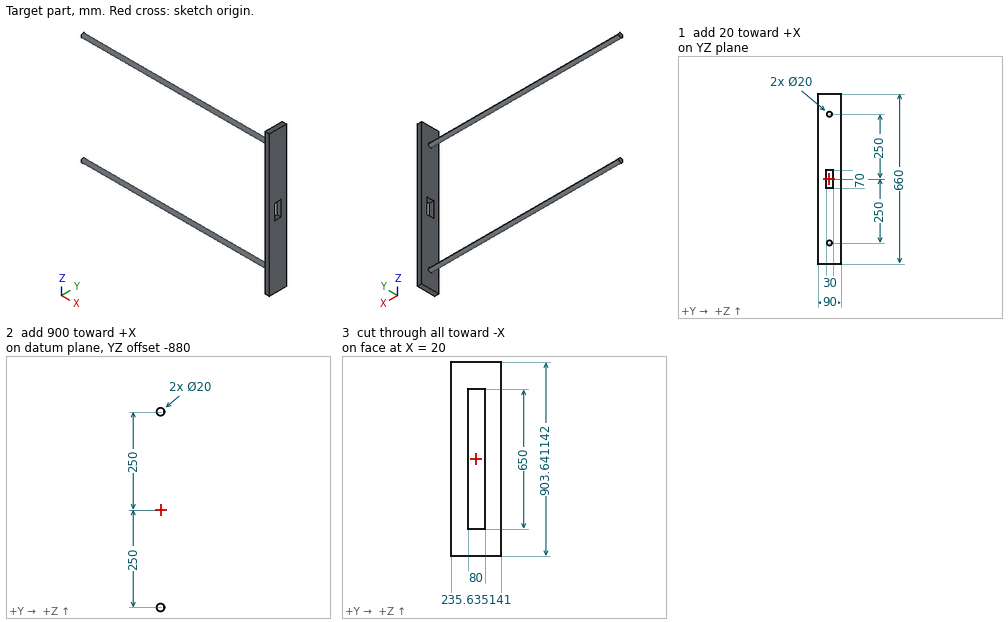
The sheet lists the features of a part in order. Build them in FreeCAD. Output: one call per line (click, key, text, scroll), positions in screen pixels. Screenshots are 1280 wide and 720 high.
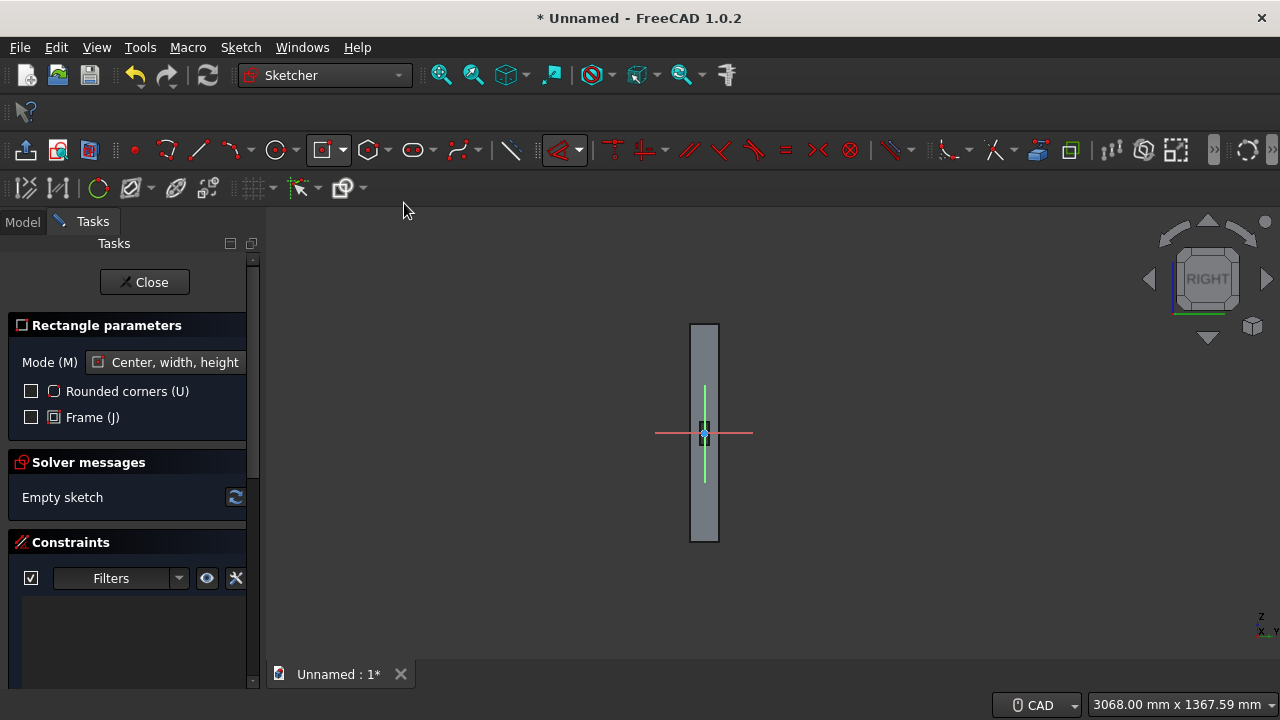
click(705, 433)
click(743, 284)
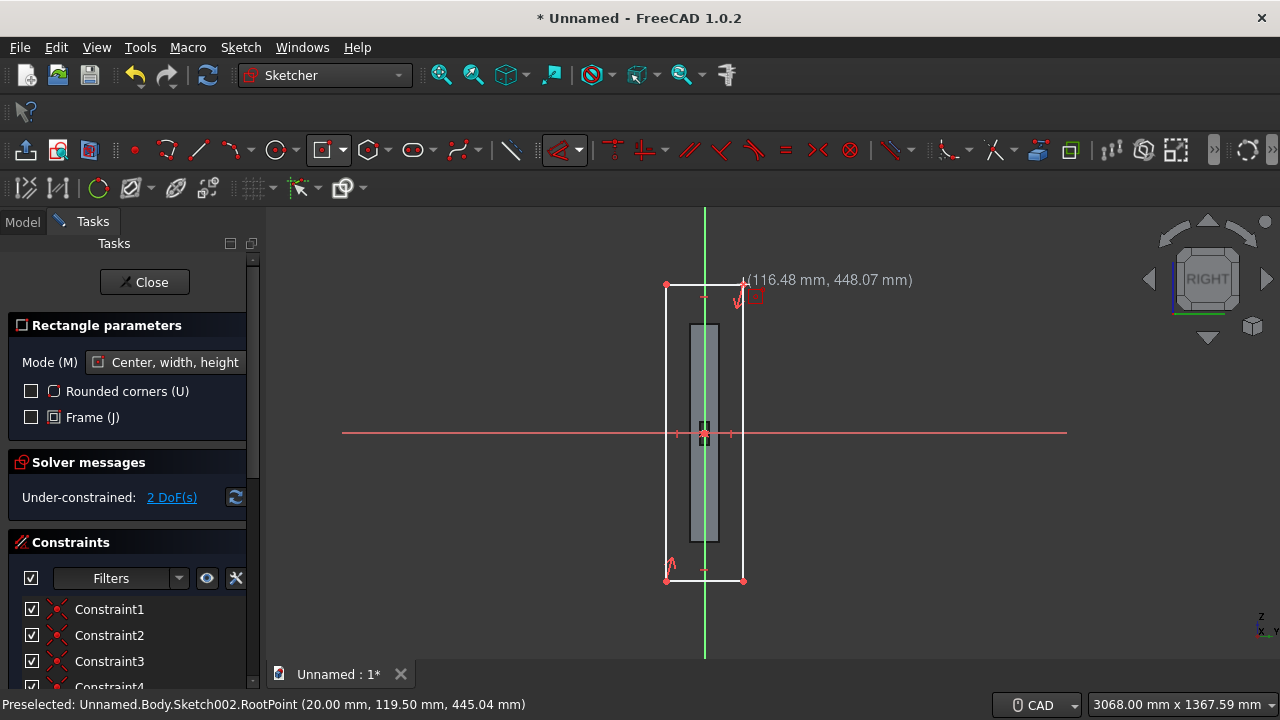
click(705, 433)
click(718, 326)
key(Escape)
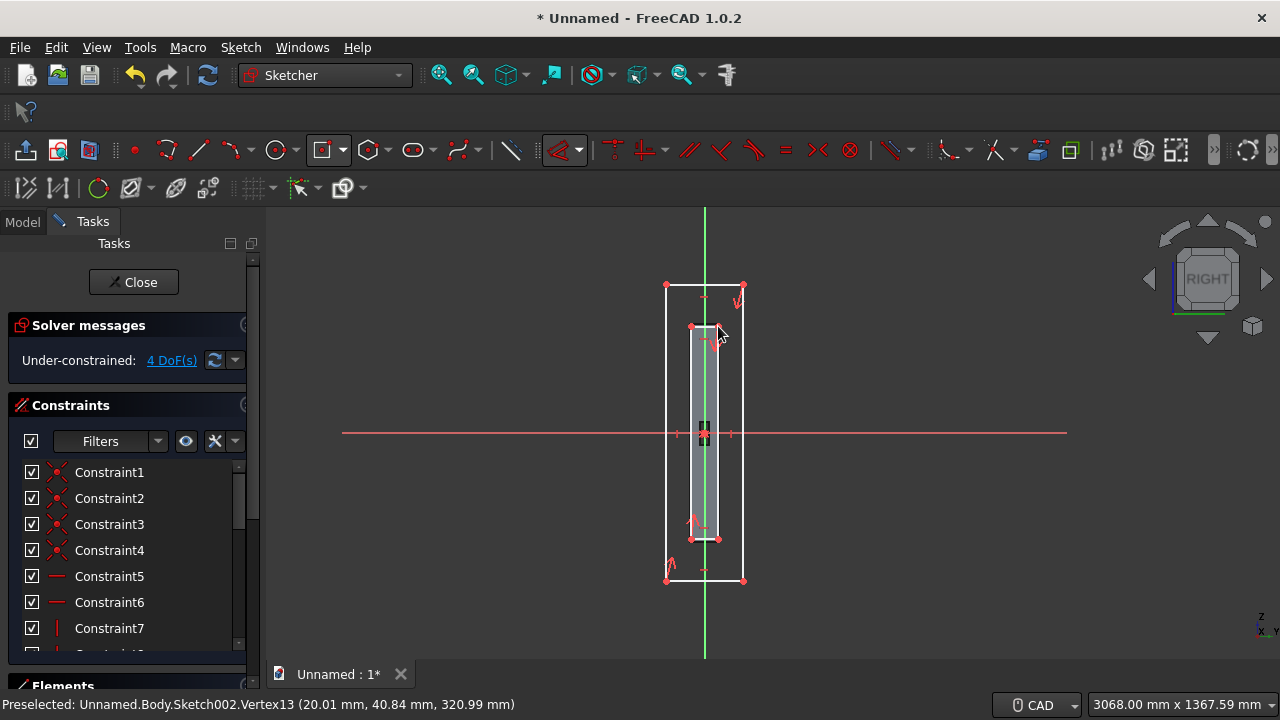
key(d)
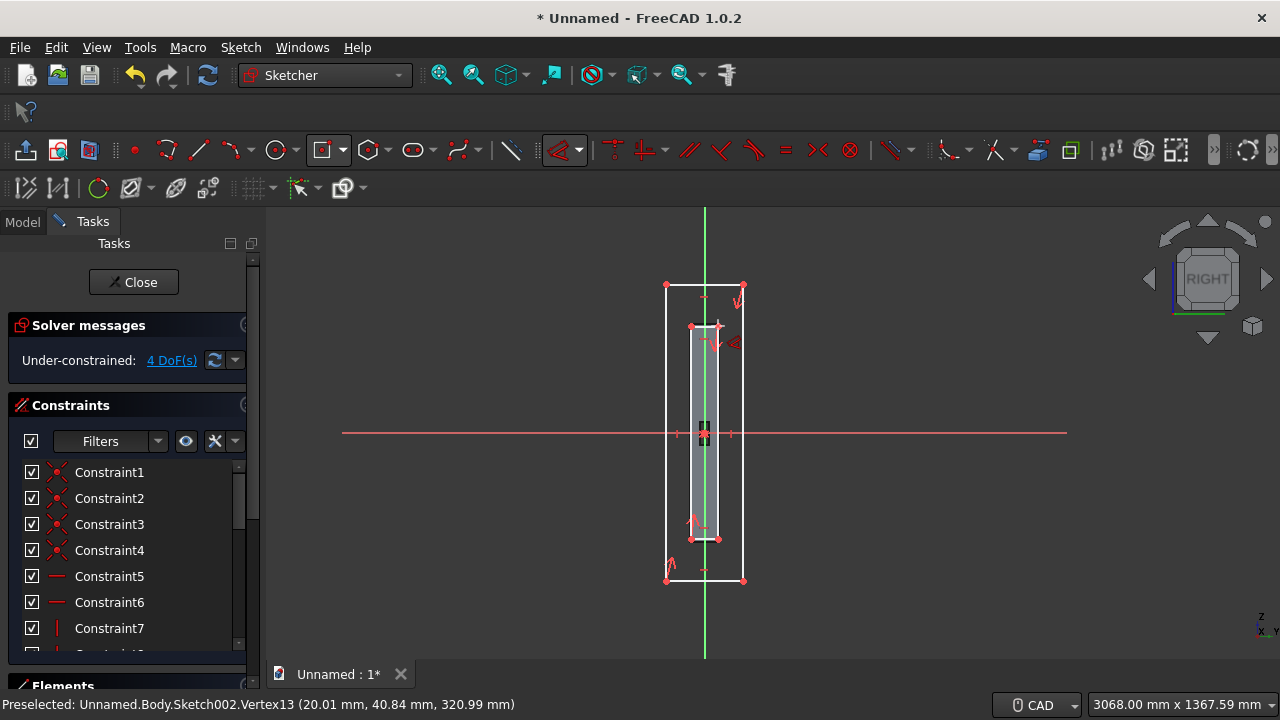
scroll(702, 539, up, 3)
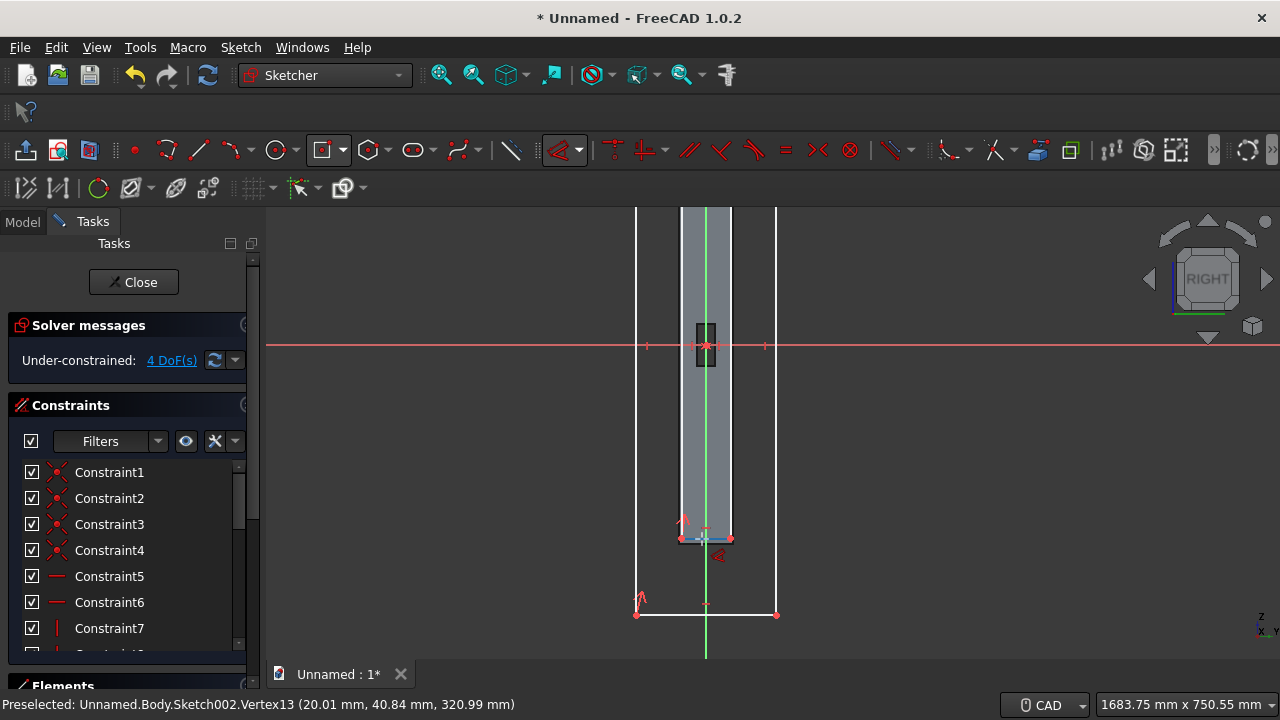
click(701, 539)
click(689, 573)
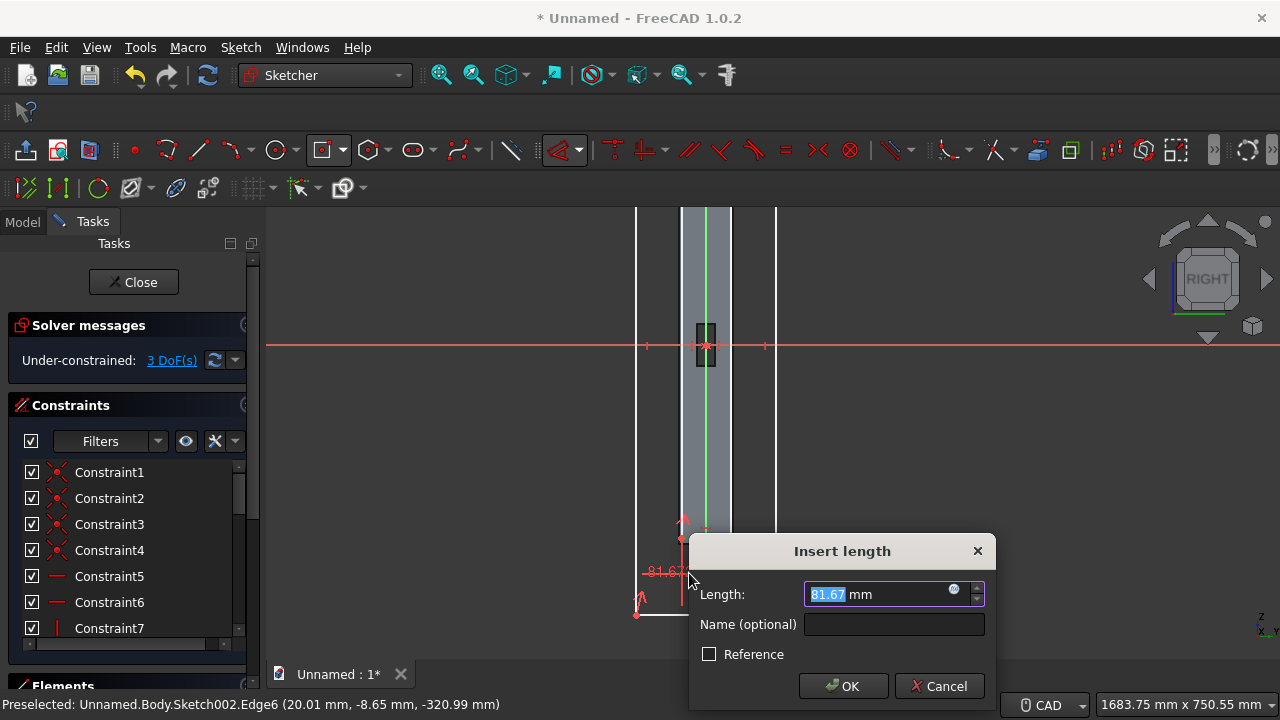
text(80)
key(Return)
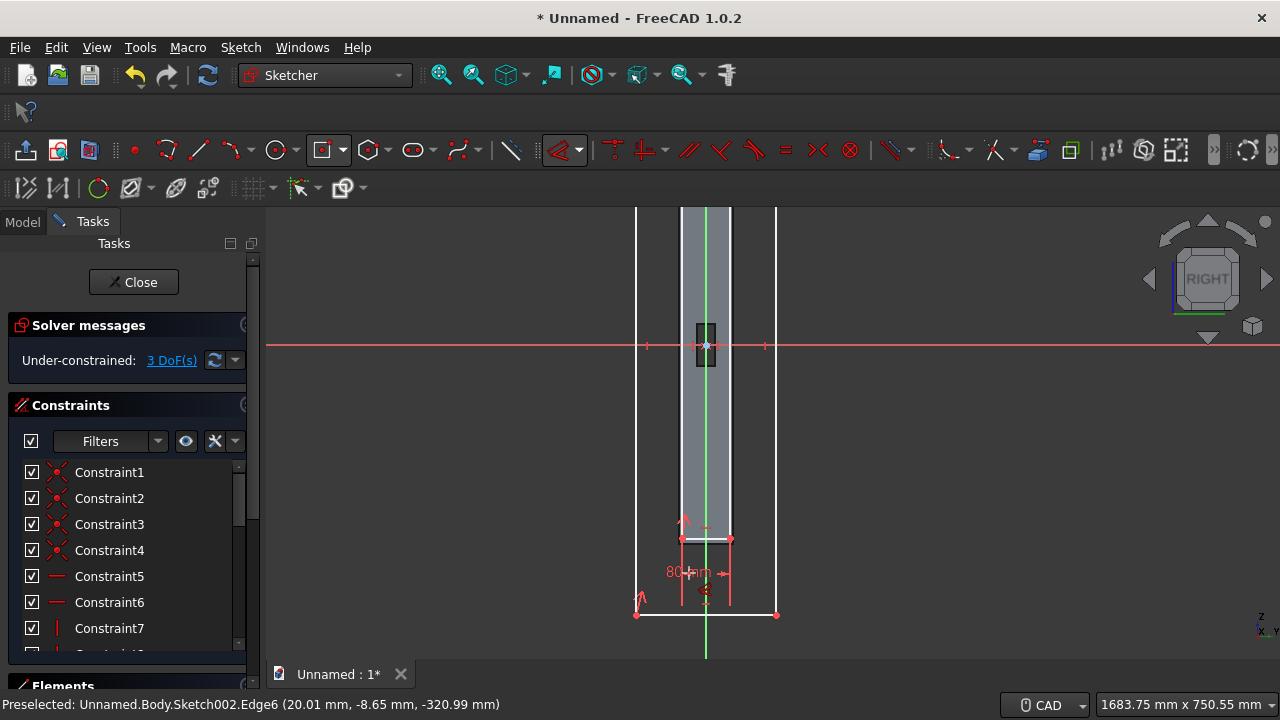
click(730, 423)
click(812, 387)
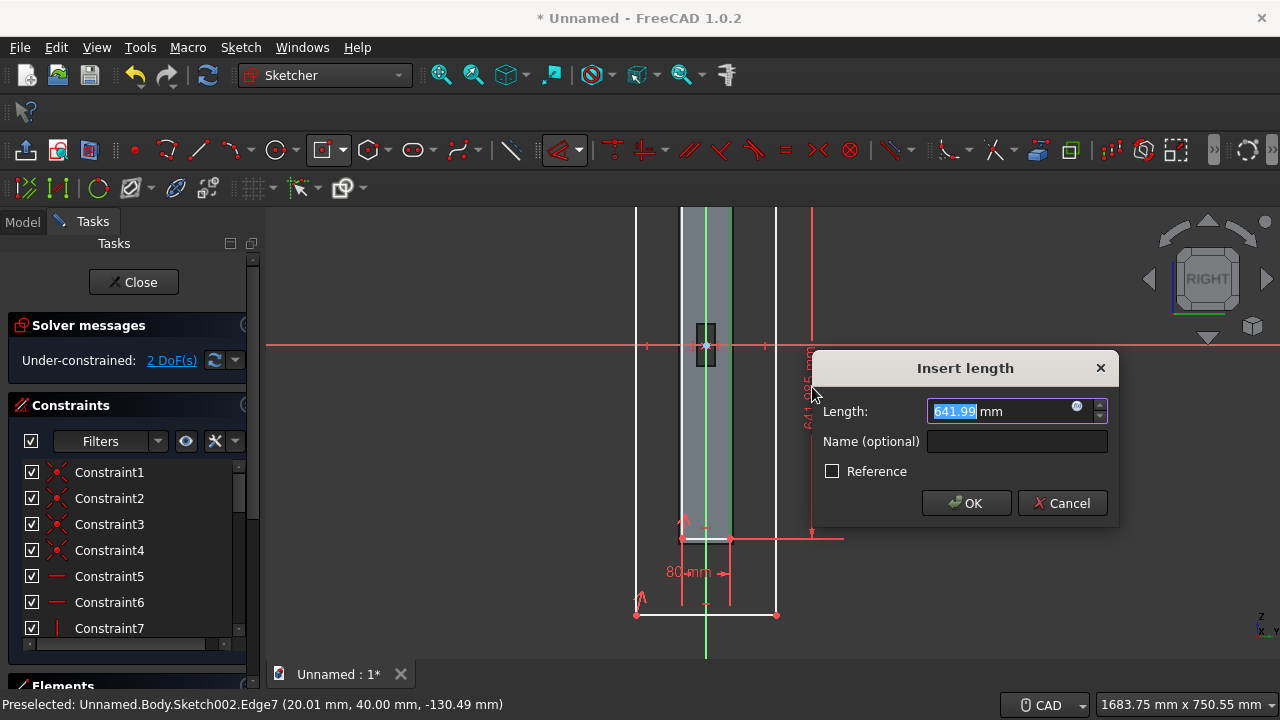
text(650)
key(Return)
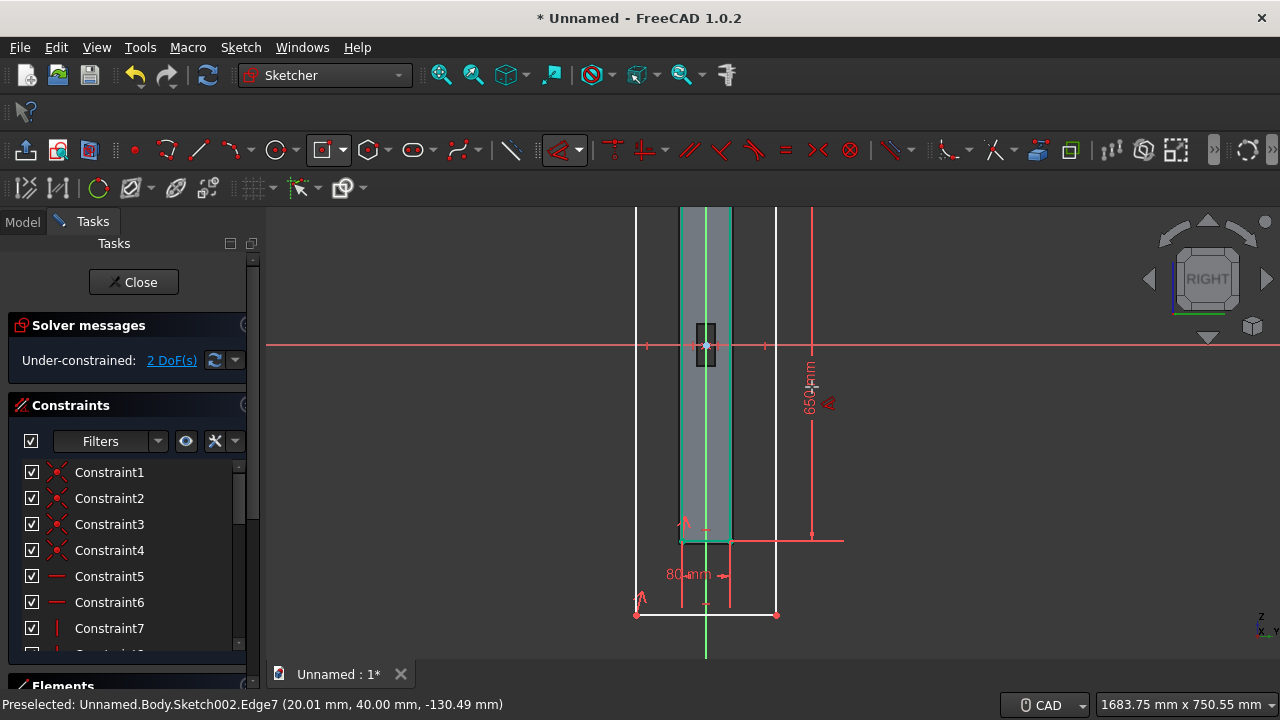
click(678, 615)
click(657, 533)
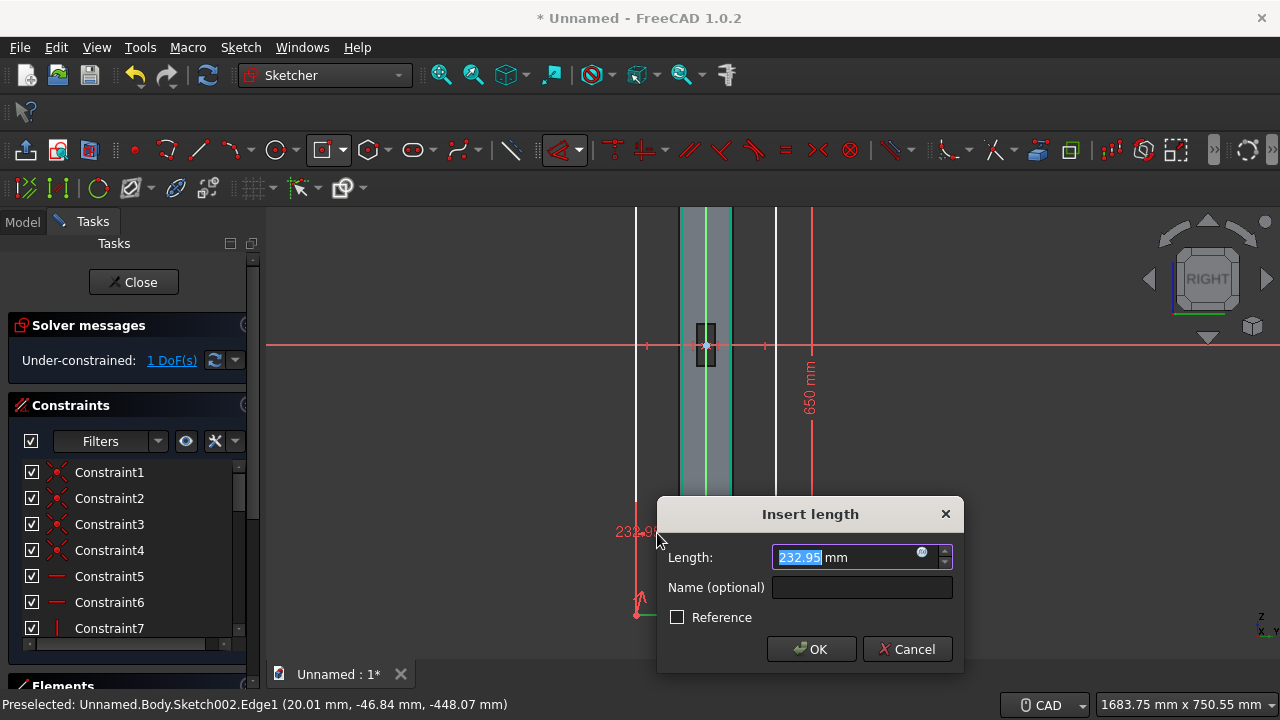
text(235.635141)
key(Return)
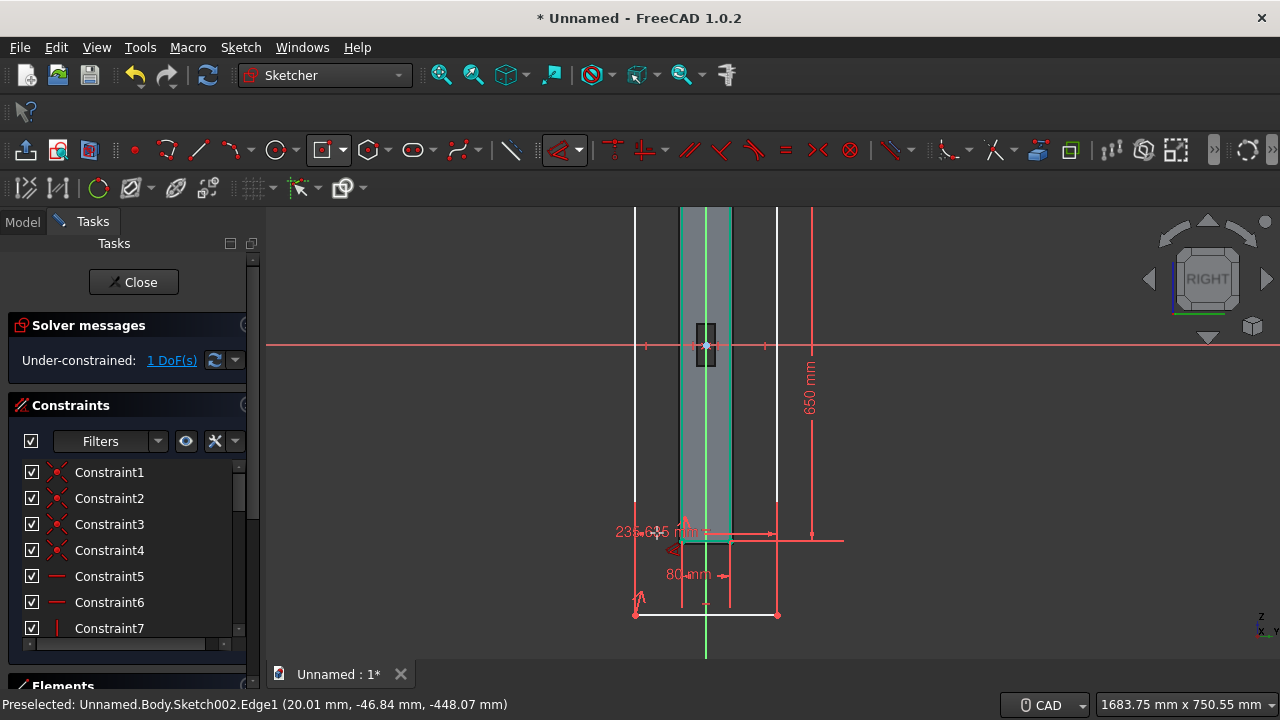
click(777, 453)
click(811, 425)